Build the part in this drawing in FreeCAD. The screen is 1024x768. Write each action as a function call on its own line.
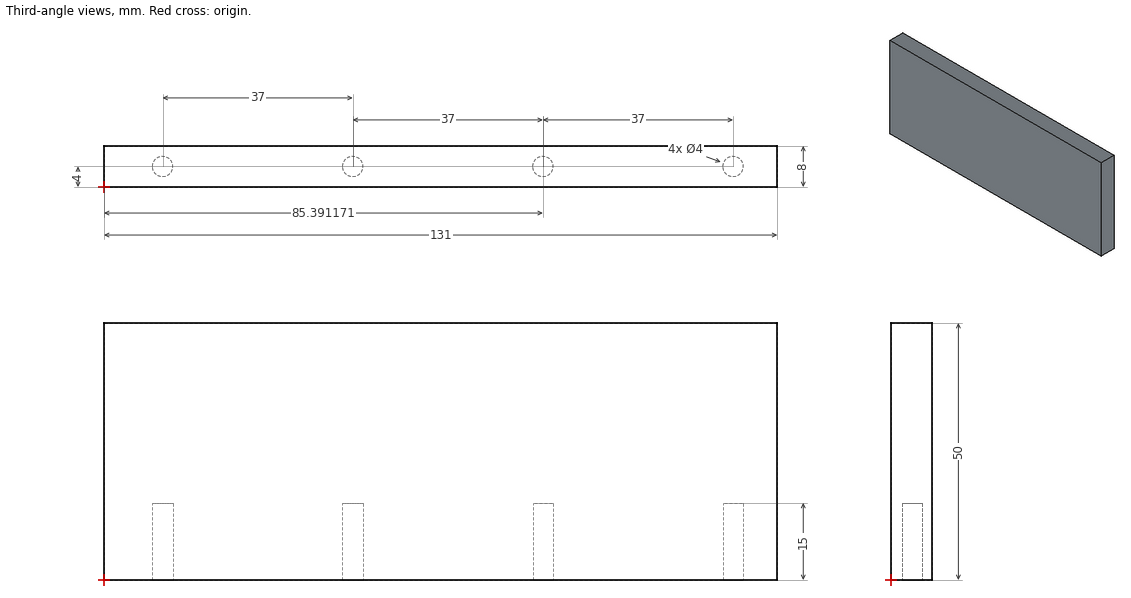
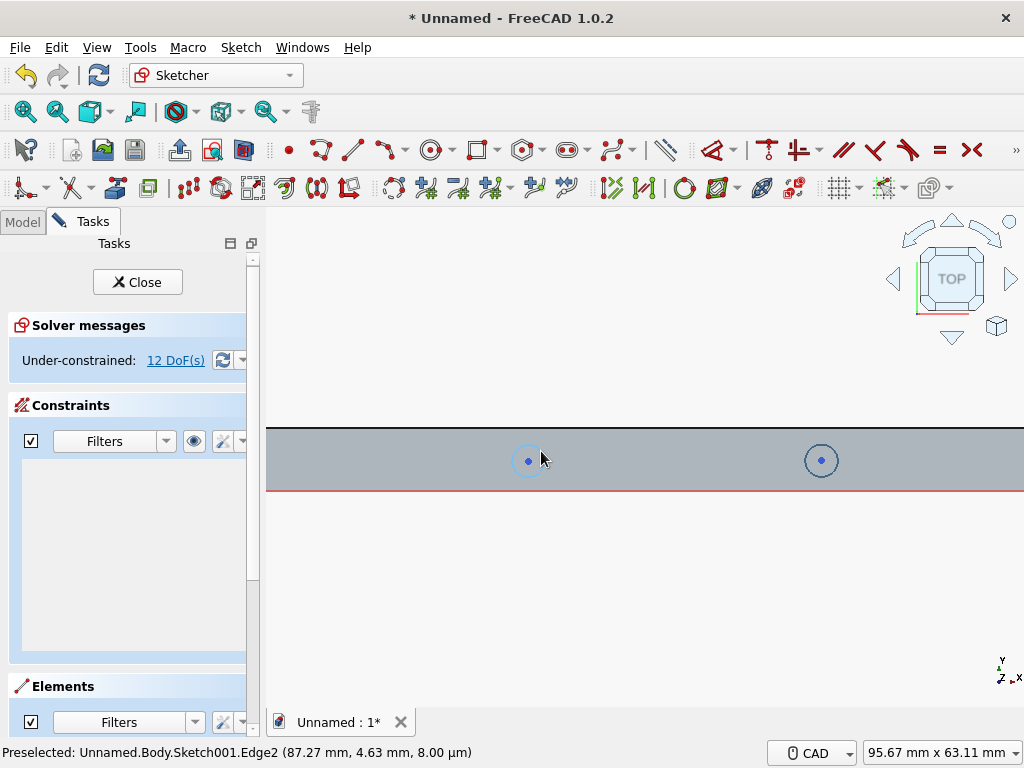
click(540, 450)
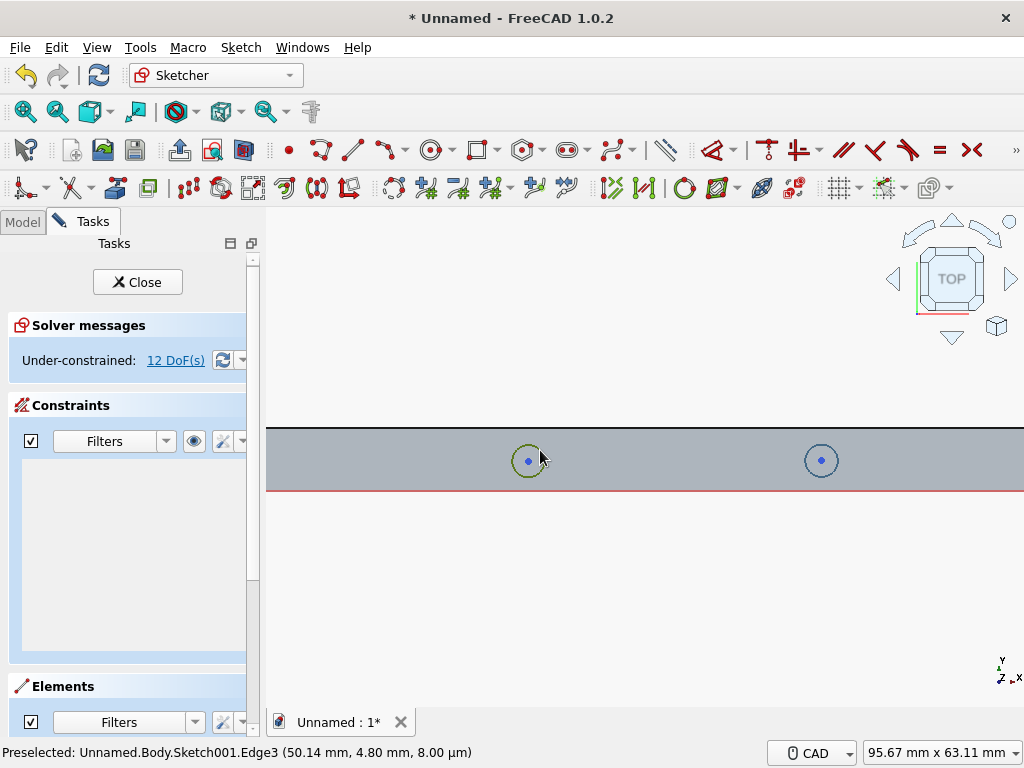
scroll(541, 451, down, 5)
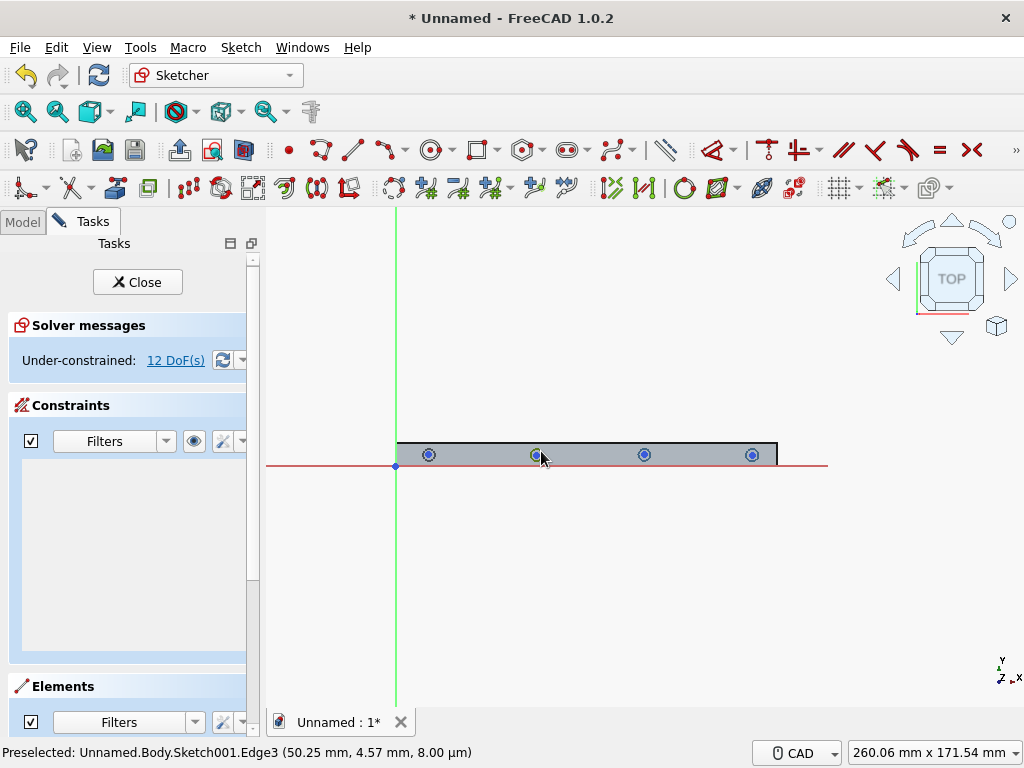
scroll(433, 451, up, 5)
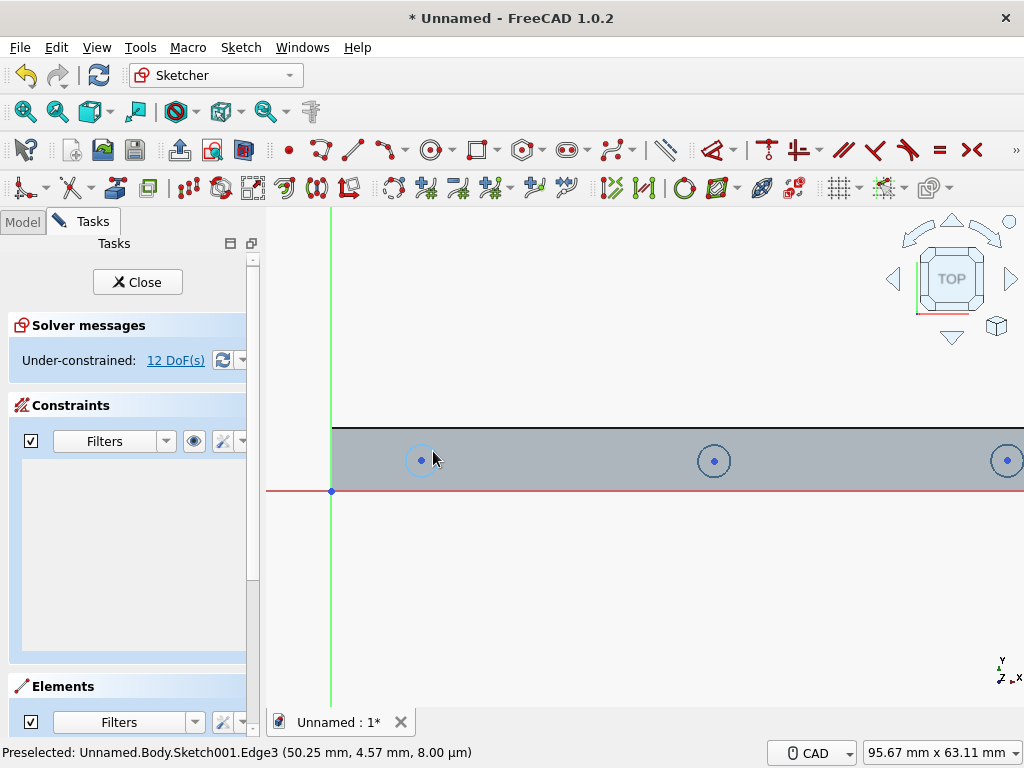
click(433, 450)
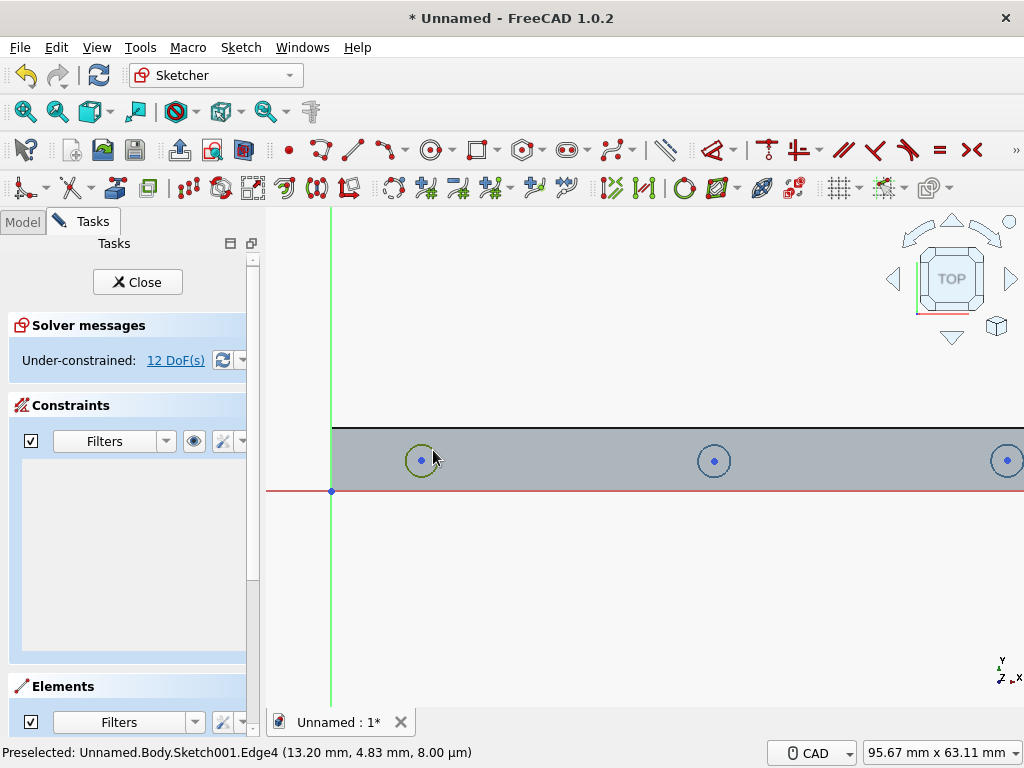
click(940, 150)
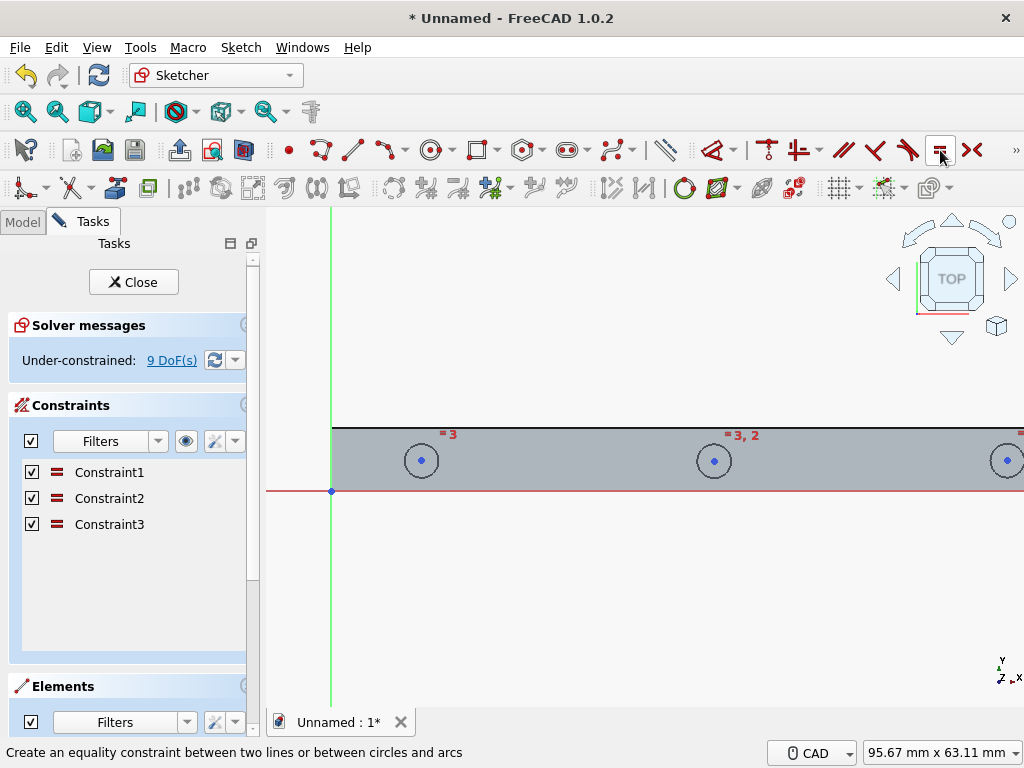
scroll(433, 451, down, 5)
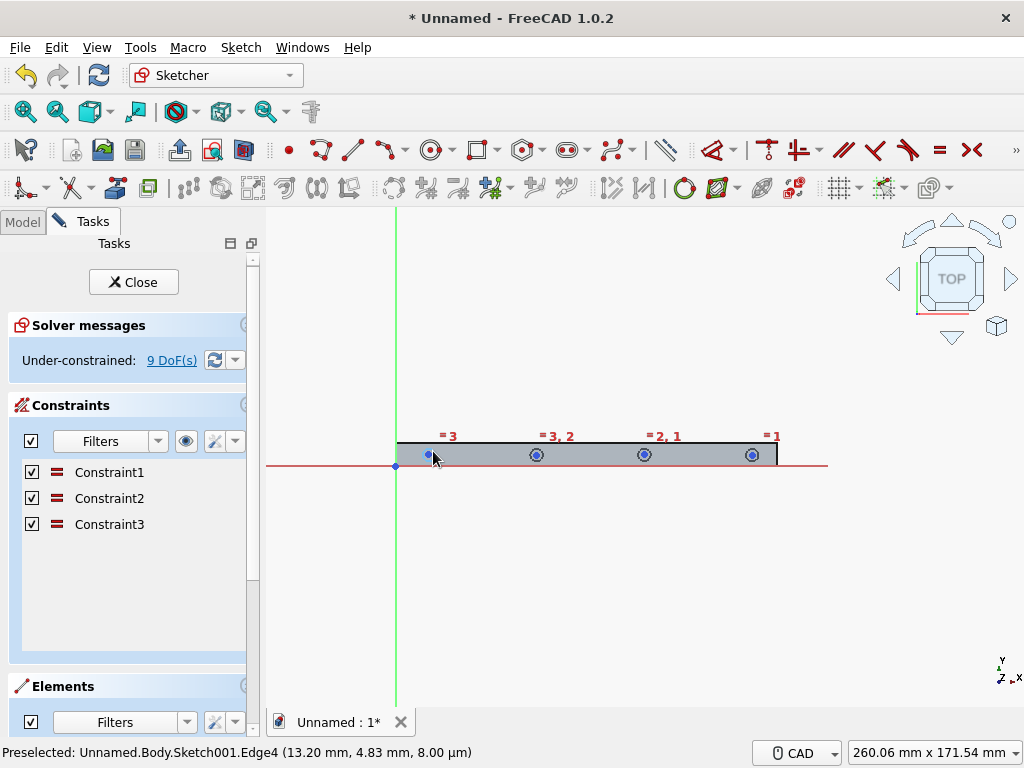
click(752, 455)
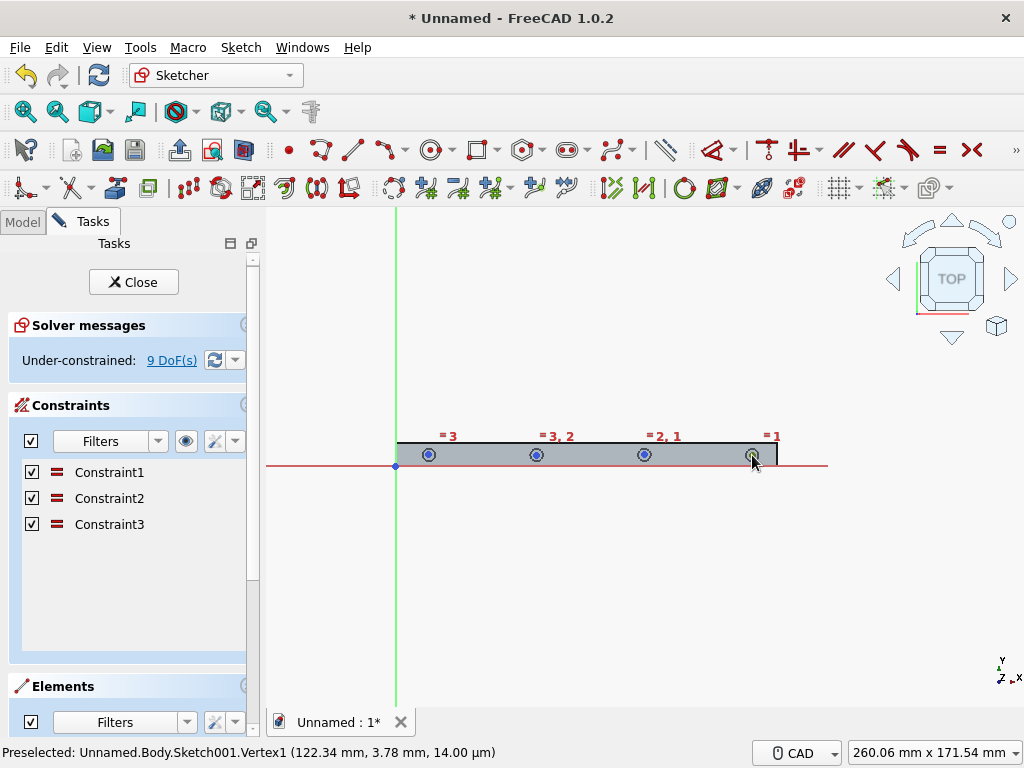
click(644, 455)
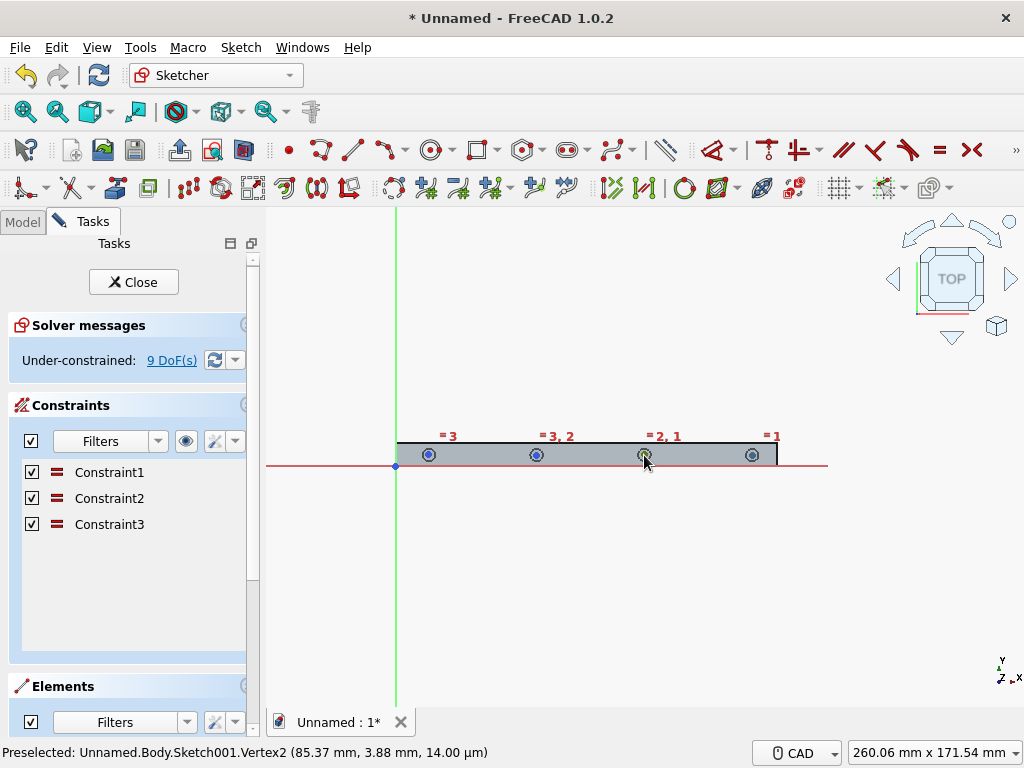
click(822, 150)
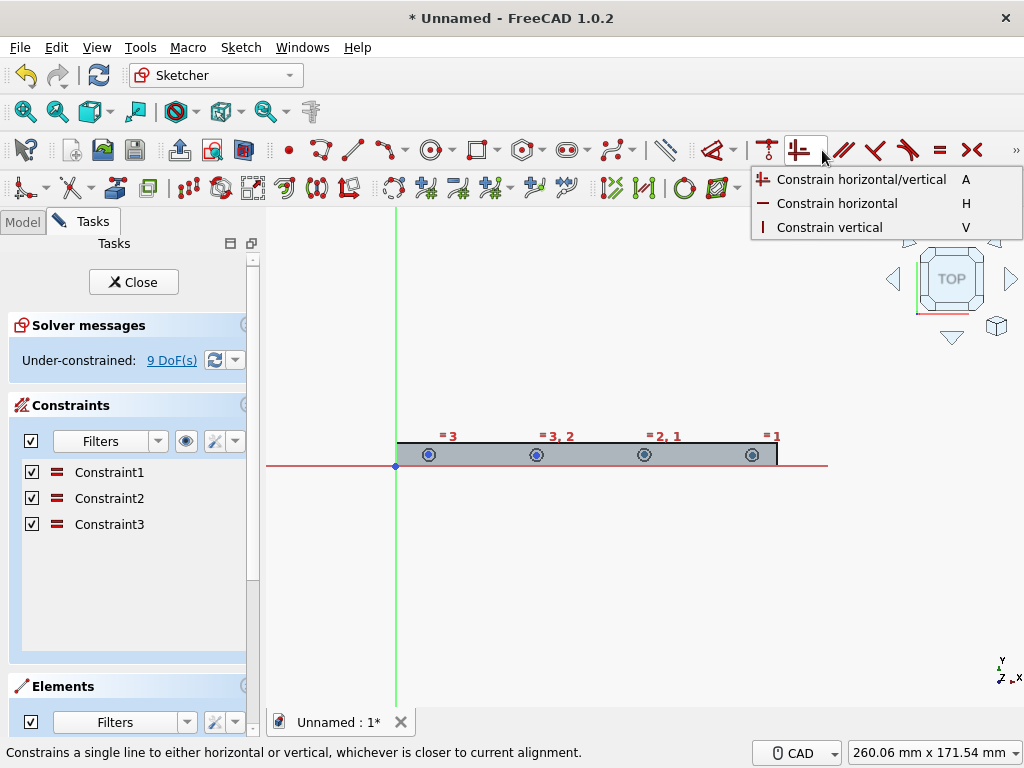
click(887, 203)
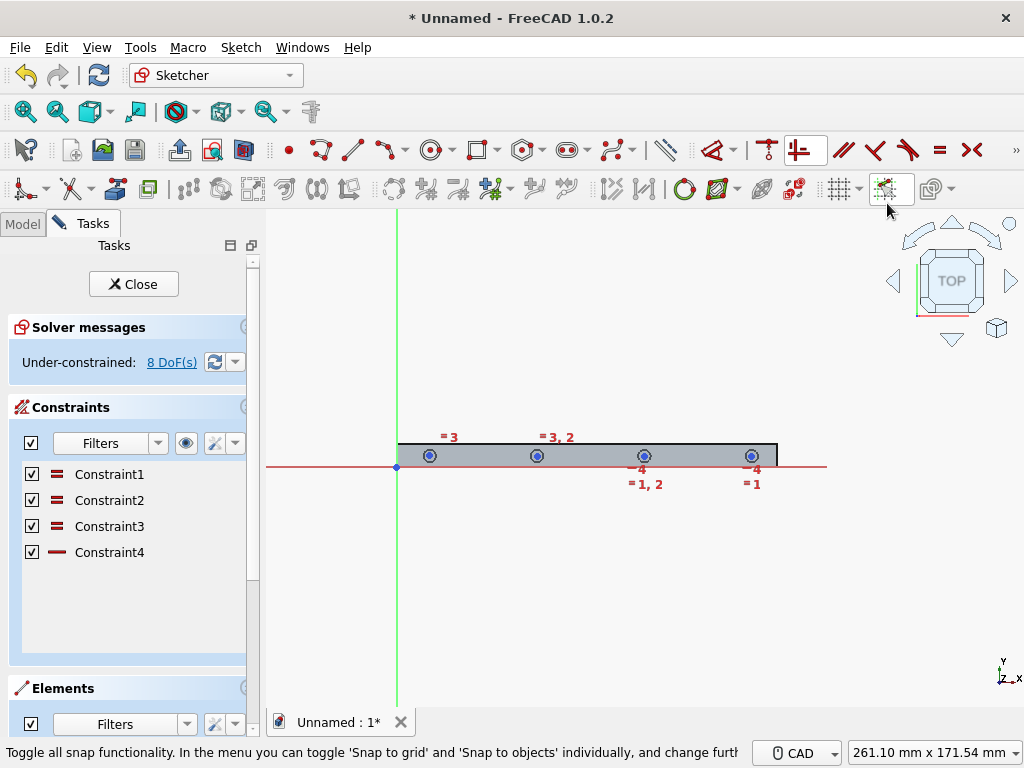
click(644, 456)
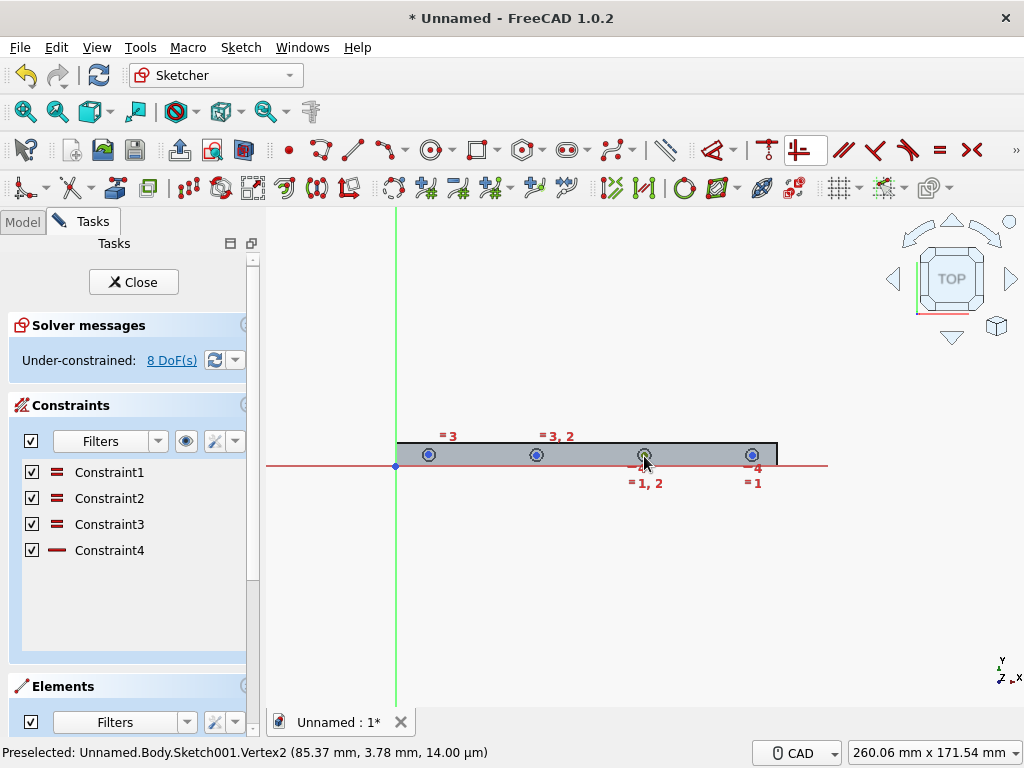
click(537, 455)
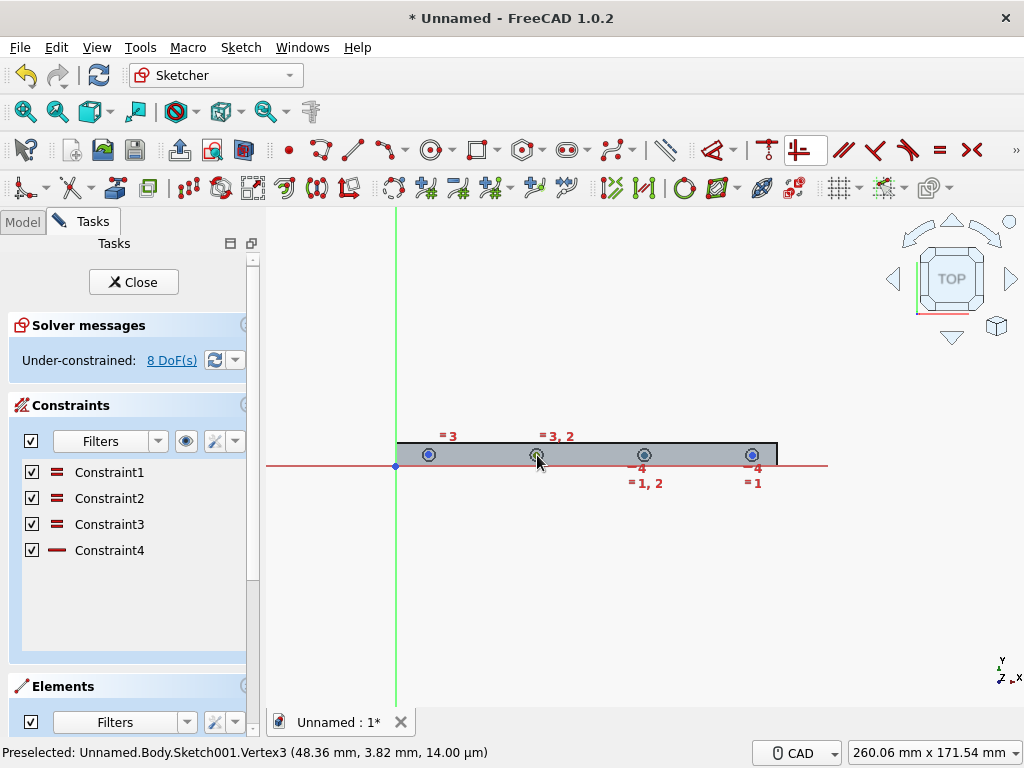
key(h)